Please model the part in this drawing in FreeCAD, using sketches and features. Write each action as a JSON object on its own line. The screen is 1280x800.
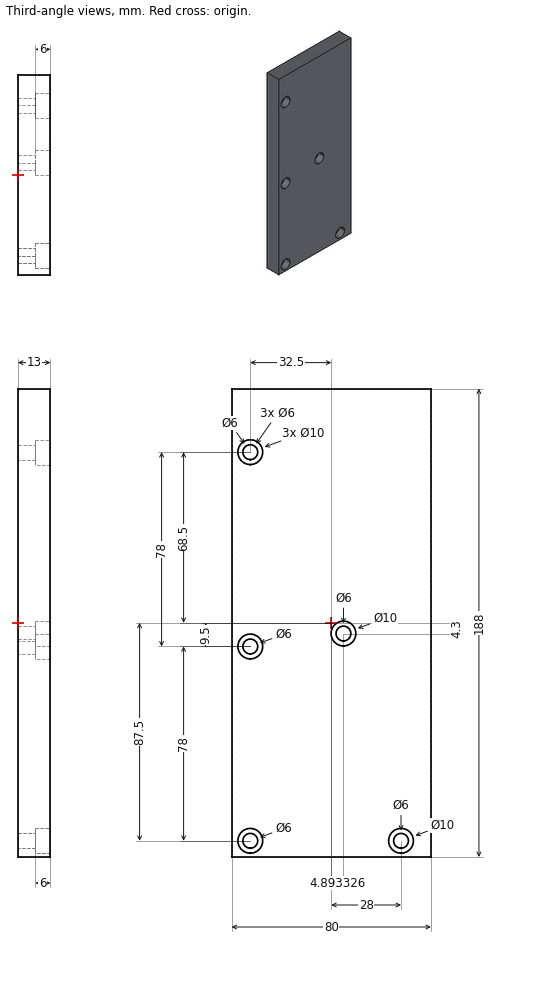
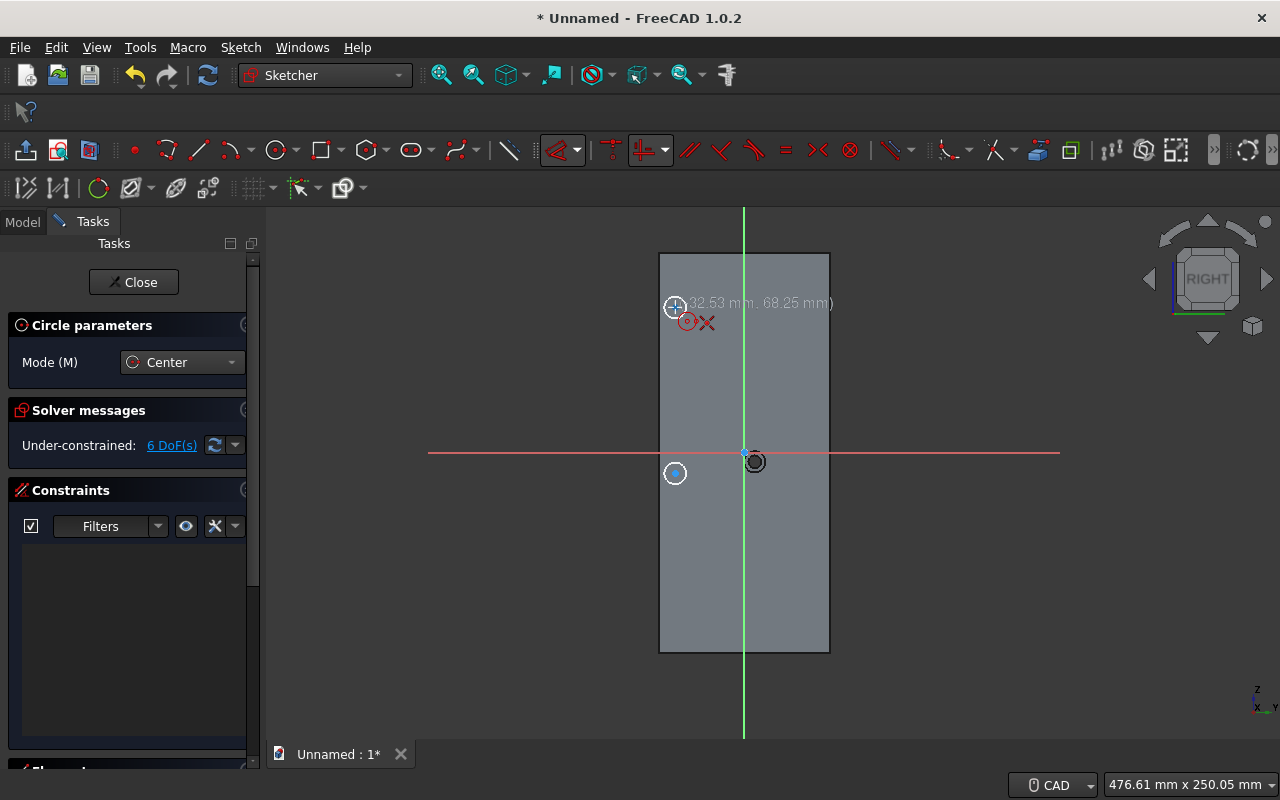
{"action": "scroll", "coordinate": [675, 639], "scroll_direction": "up", "scroll_amount": 4}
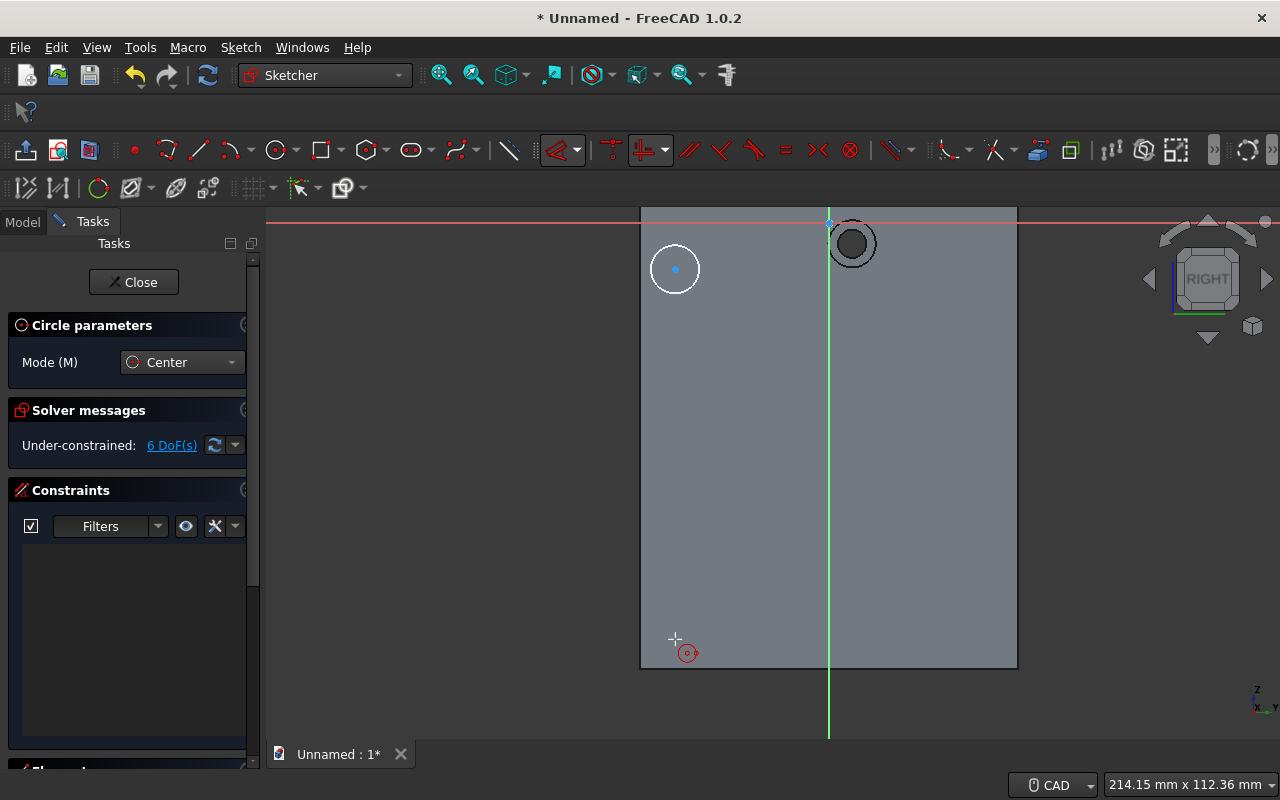
{"action": "left_click", "coordinate": [675, 638]}
{"action": "left_click", "coordinate": [692, 621]}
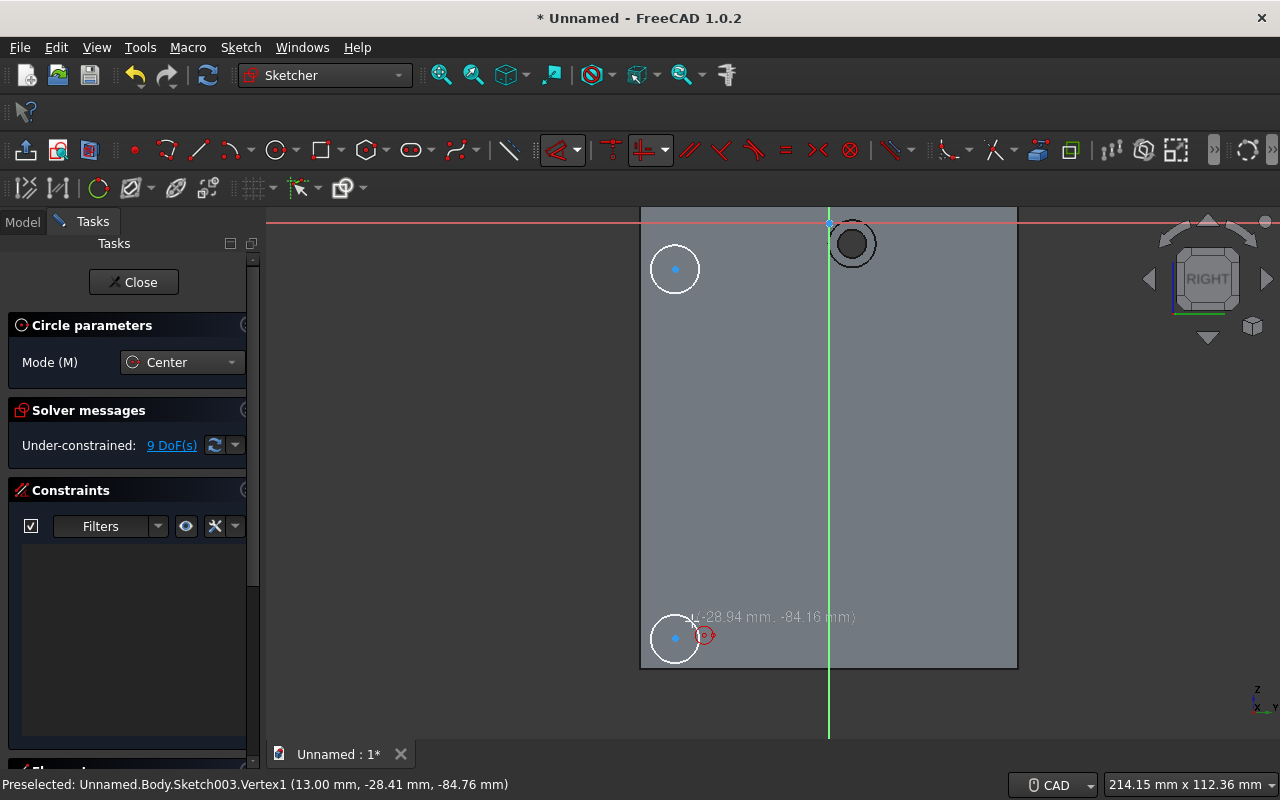
{"action": "scroll", "coordinate": [675, 640], "scroll_direction": "down", "scroll_amount": 4}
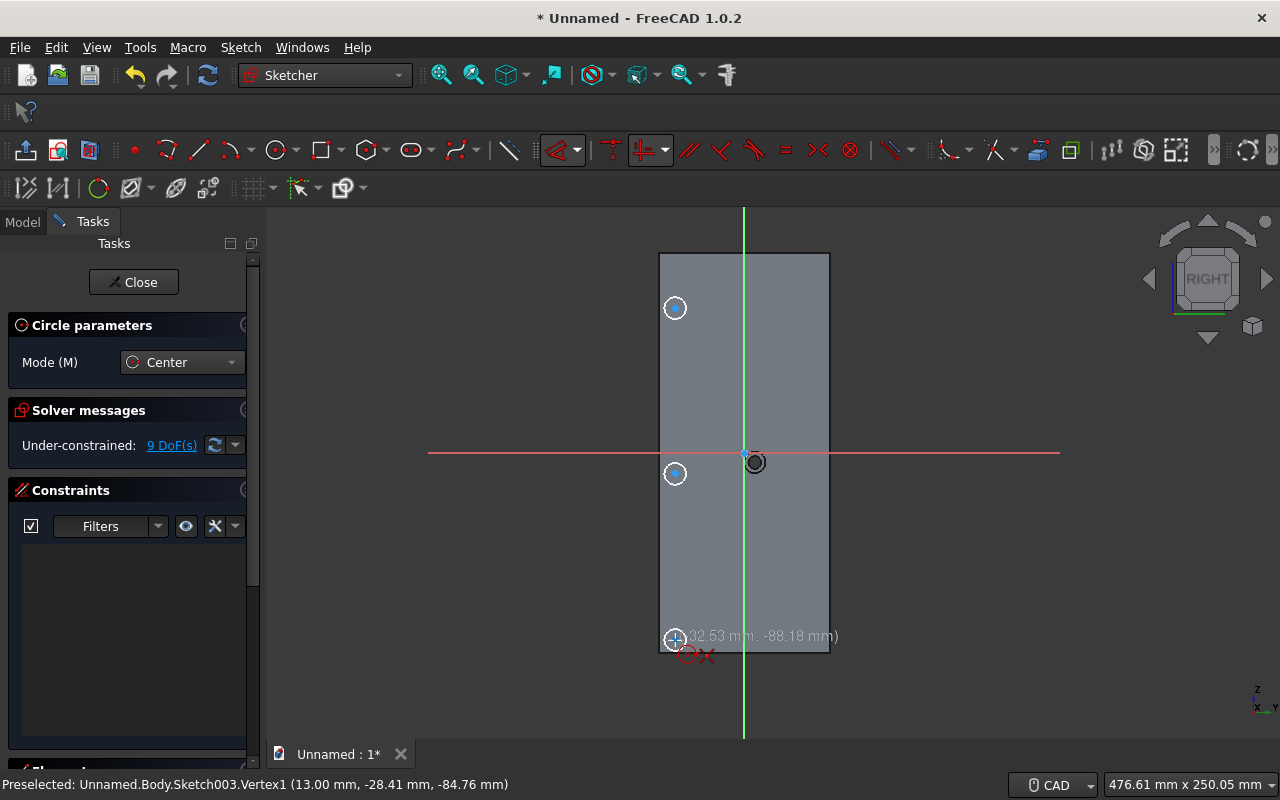
{"action": "scroll", "coordinate": [675, 308], "scroll_direction": "up", "scroll_amount": 7}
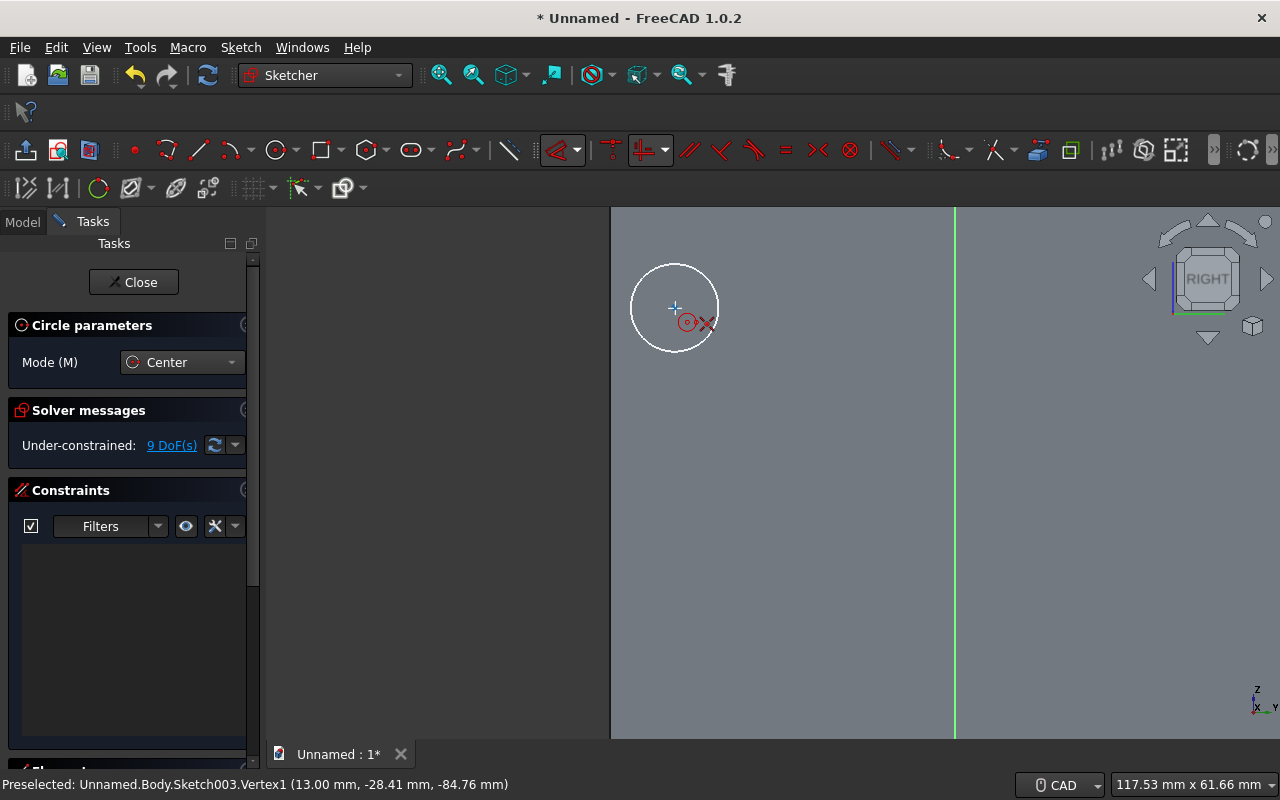
{"action": "left_click", "coordinate": [675, 308]}
{"action": "left_click", "coordinate": [693, 287]}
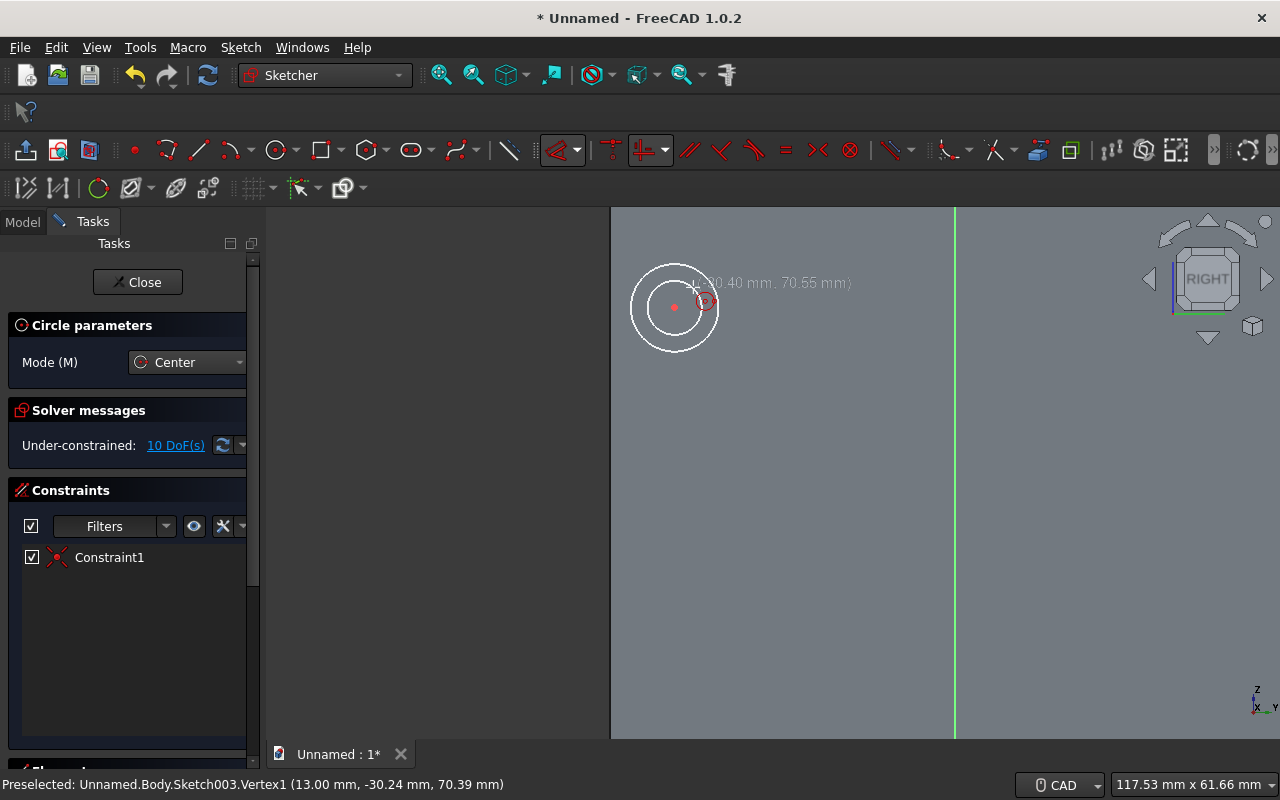
{"action": "scroll", "coordinate": [675, 308], "scroll_direction": "down", "scroll_amount": 7}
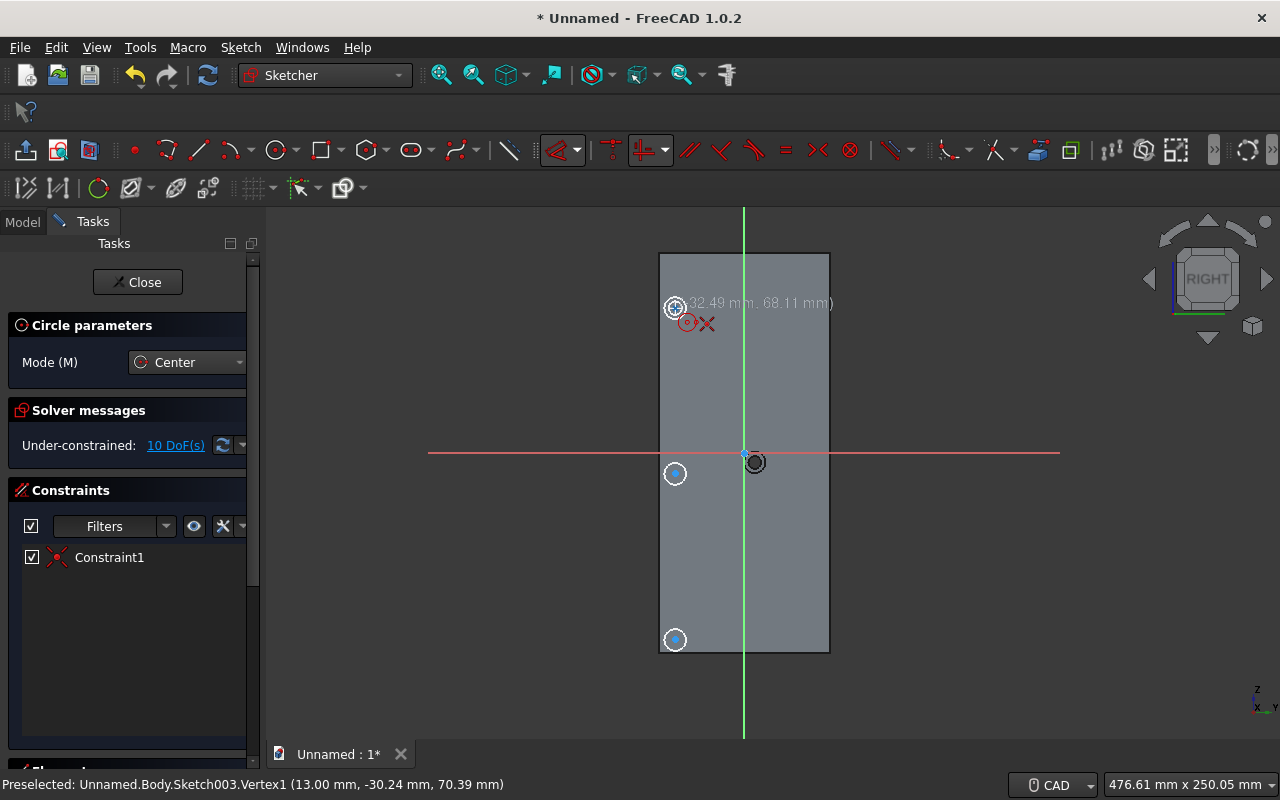
{"action": "scroll", "coordinate": [675, 474], "scroll_direction": "up", "scroll_amount": 7}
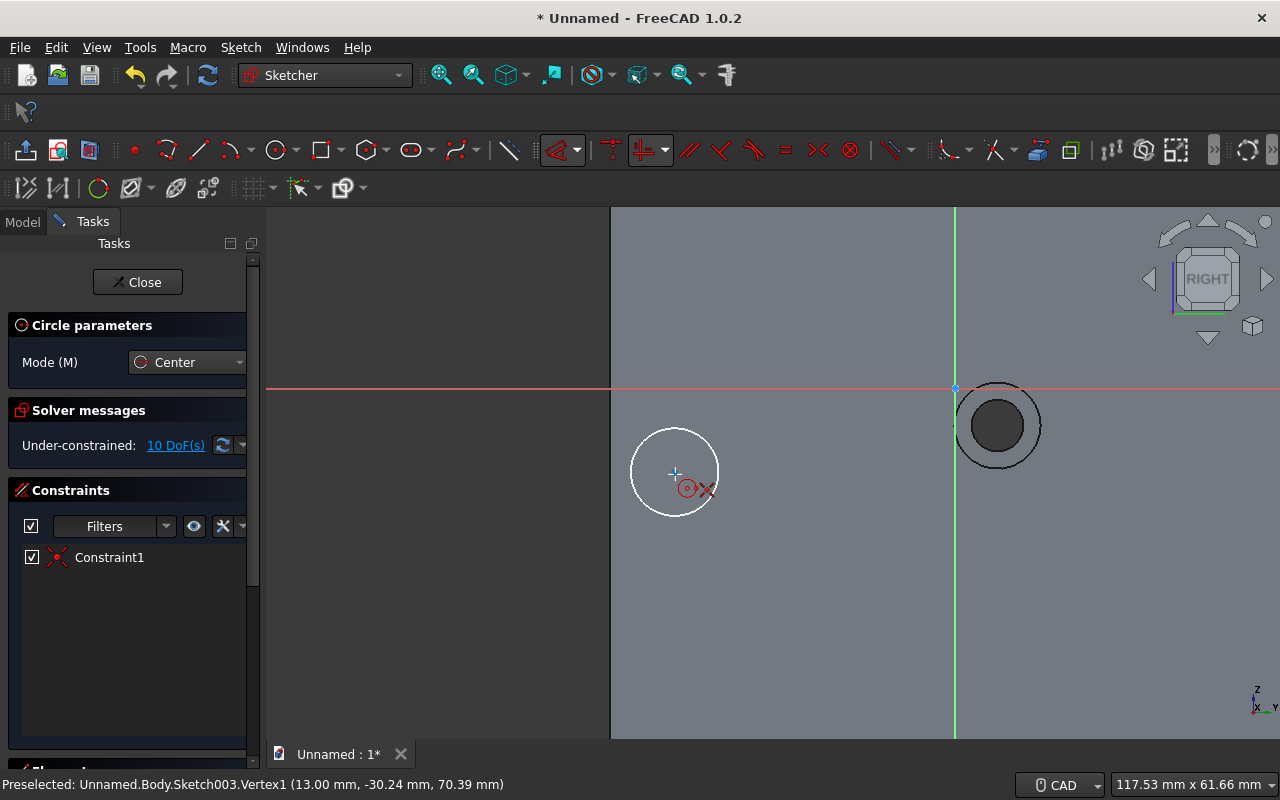
{"action": "left_click", "coordinate": [675, 472]}
{"action": "left_click", "coordinate": [693, 452]}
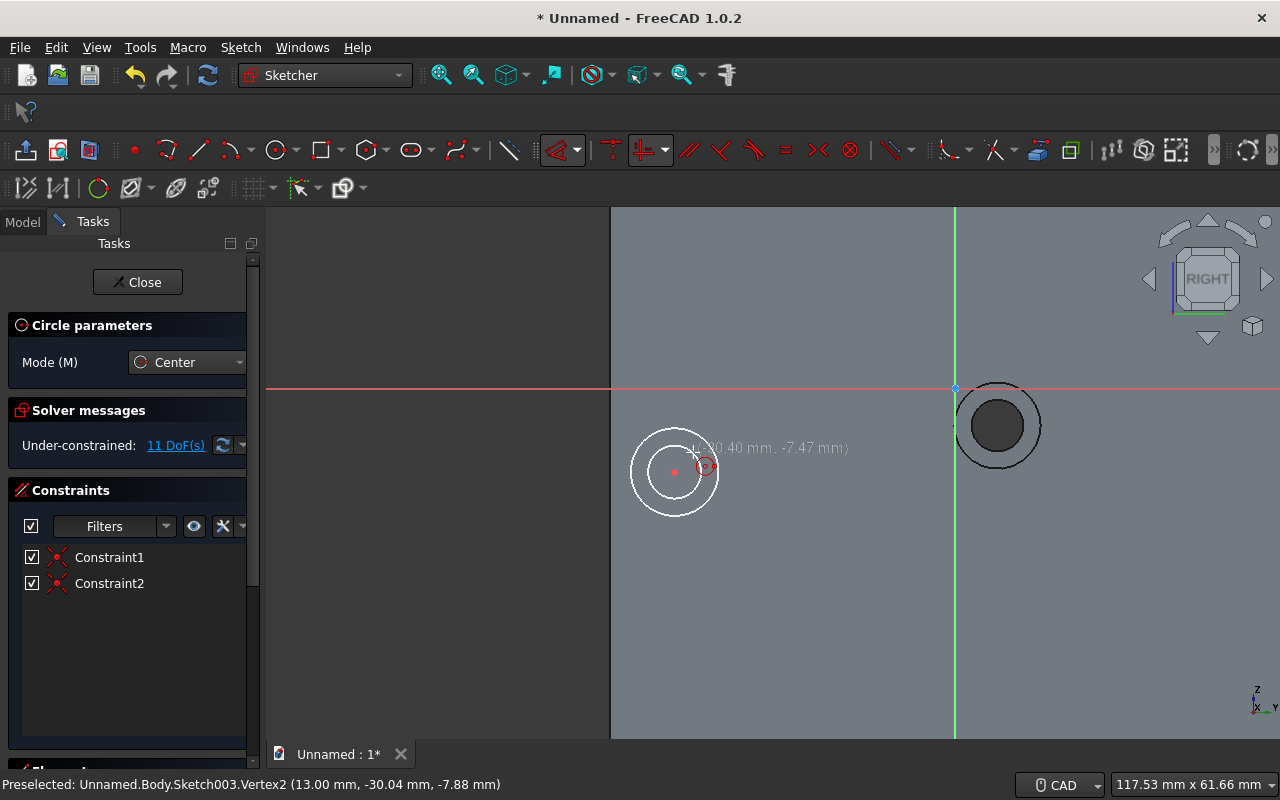
{"action": "scroll", "coordinate": [675, 474], "scroll_direction": "down", "scroll_amount": 7}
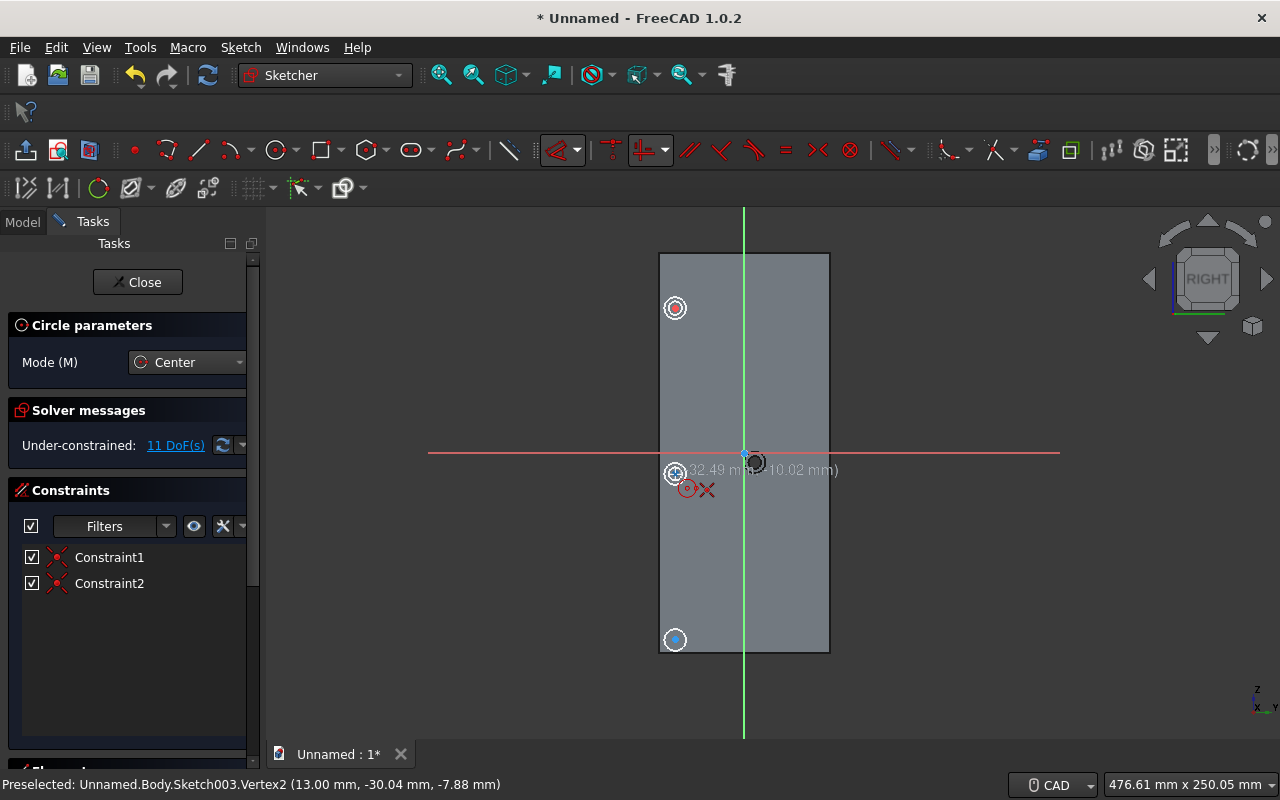
{"action": "scroll", "coordinate": [675, 639], "scroll_direction": "up", "scroll_amount": 7}